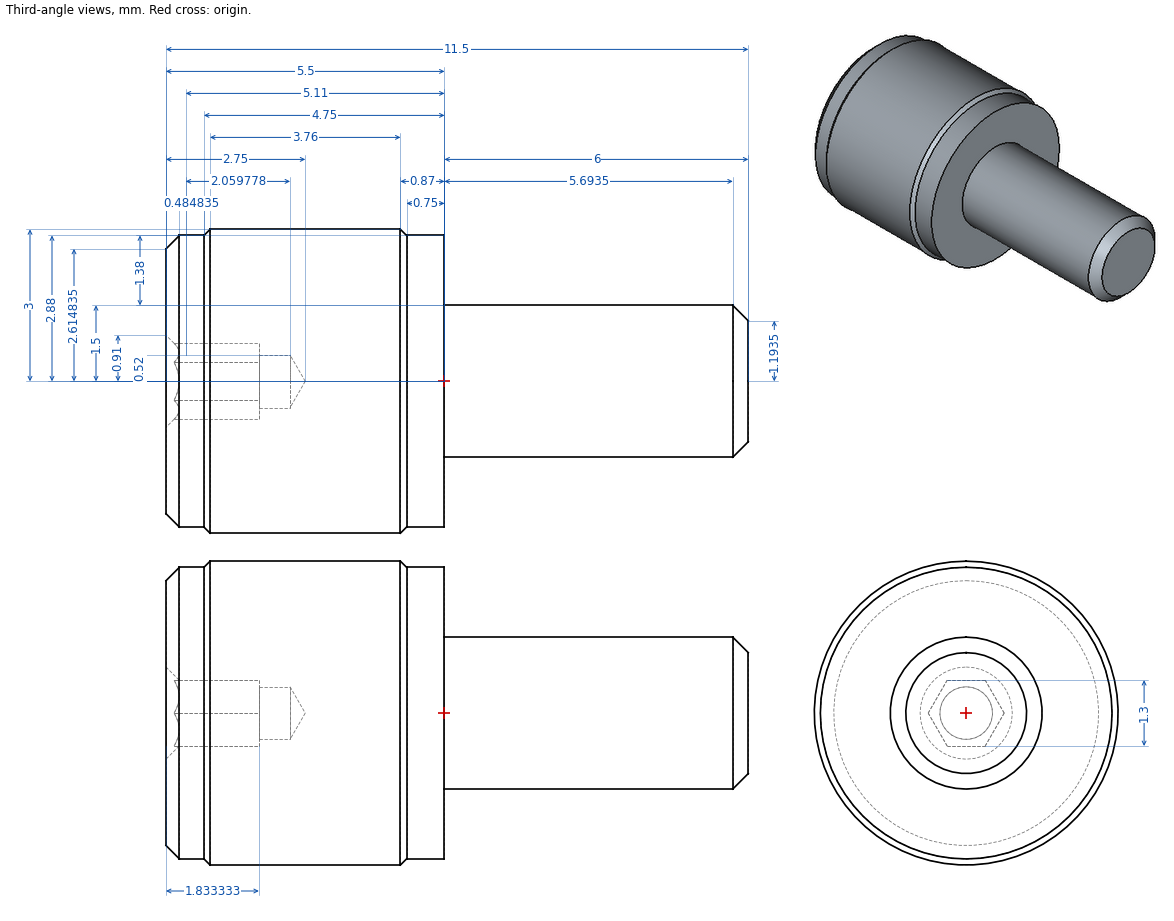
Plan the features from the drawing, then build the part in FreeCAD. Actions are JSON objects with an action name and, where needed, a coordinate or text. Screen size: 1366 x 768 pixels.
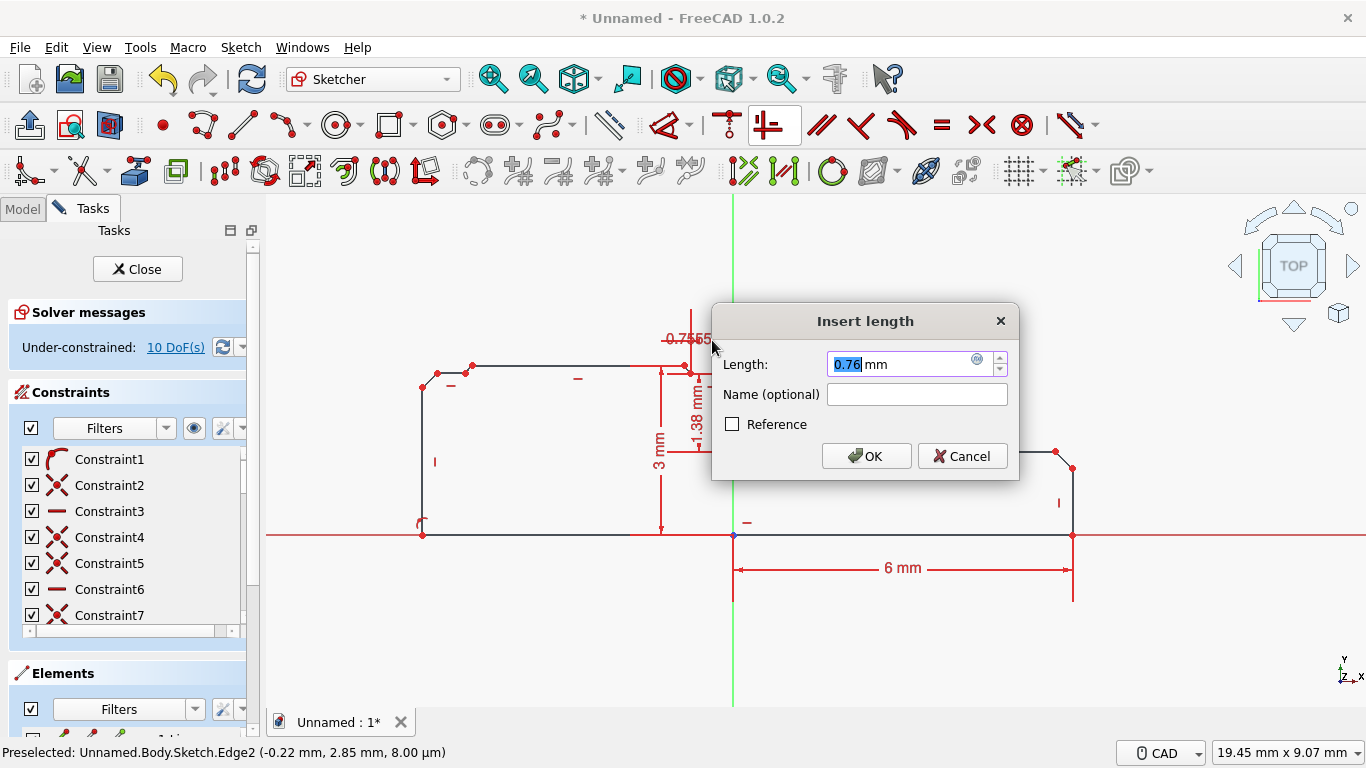
{"action": "type", "text": "0.75"}
{"action": "key", "text": "Return"}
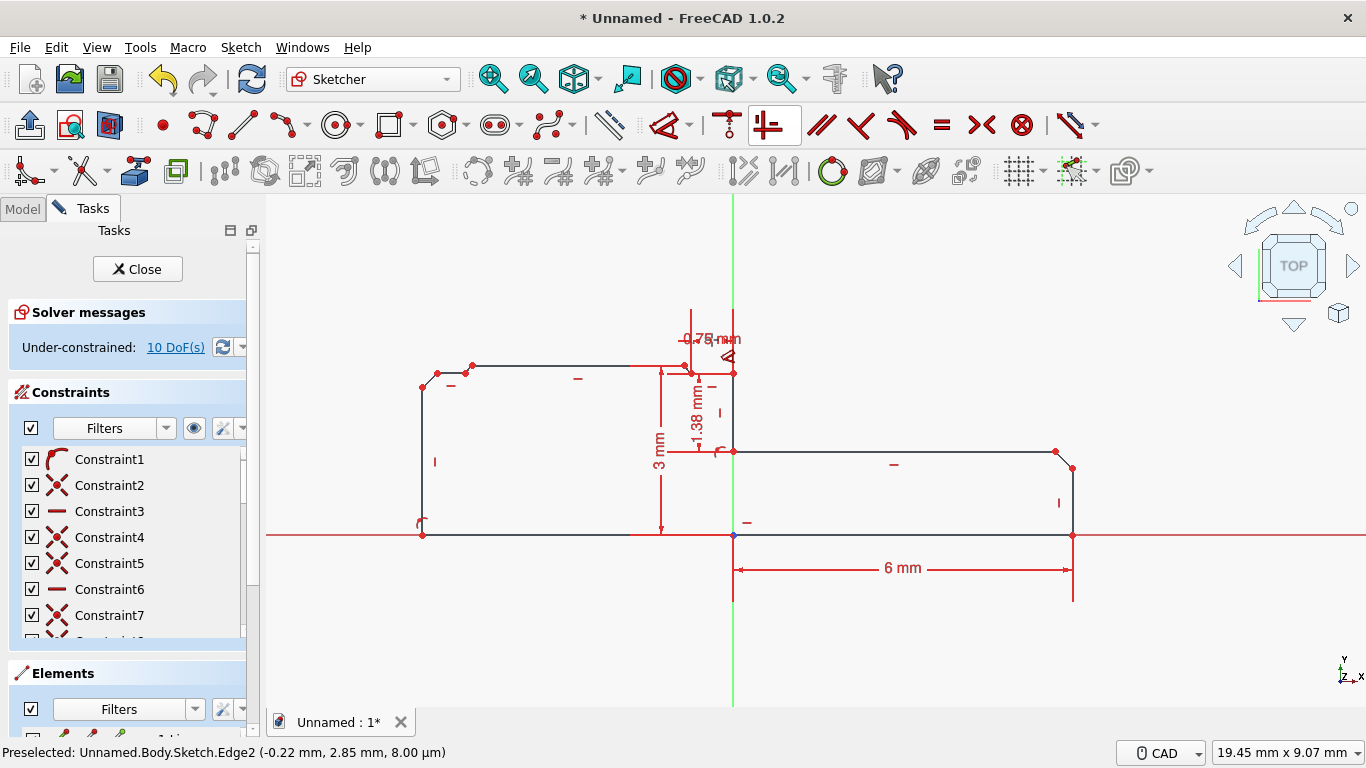
{"action": "left_click", "coordinate": [621, 366]}
{"action": "left_click", "coordinate": [578, 332]}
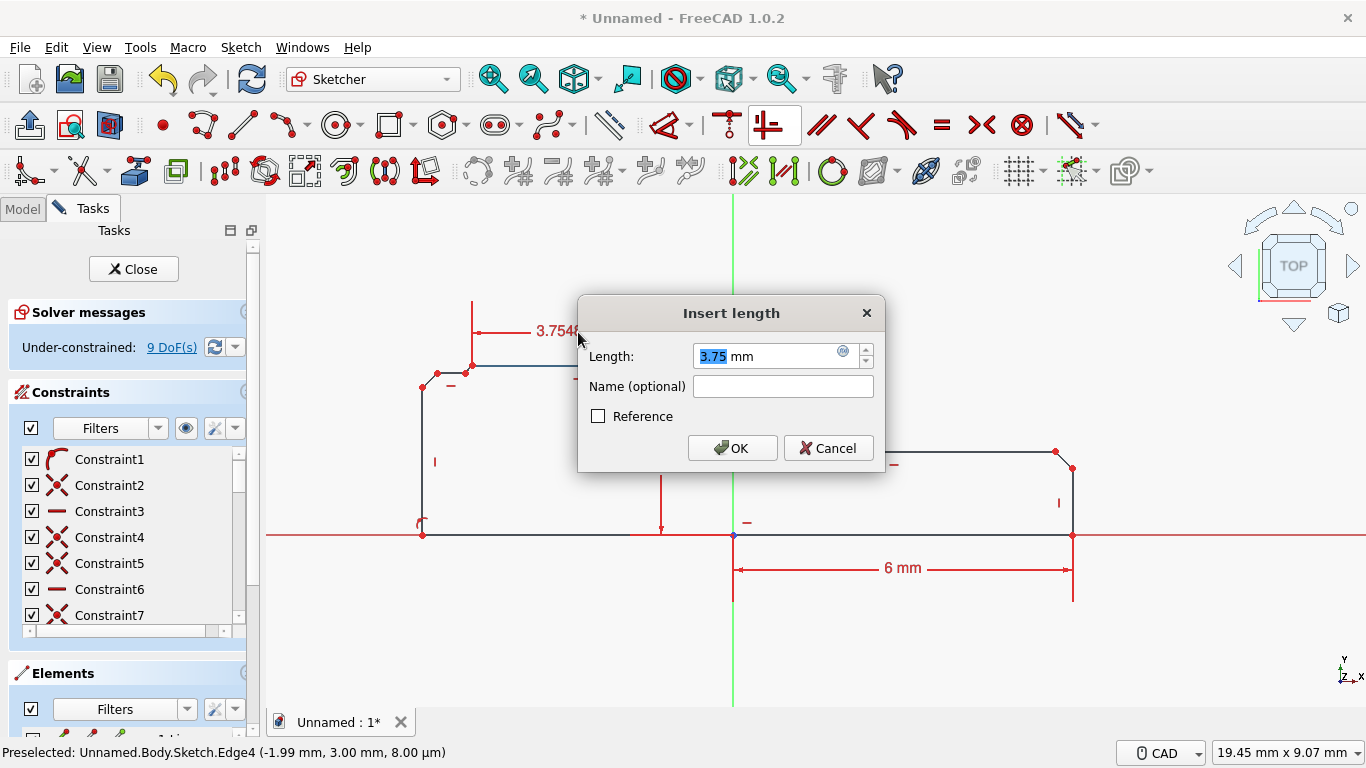
{"action": "type", "text": "3.76"}
{"action": "key", "text": "Return"}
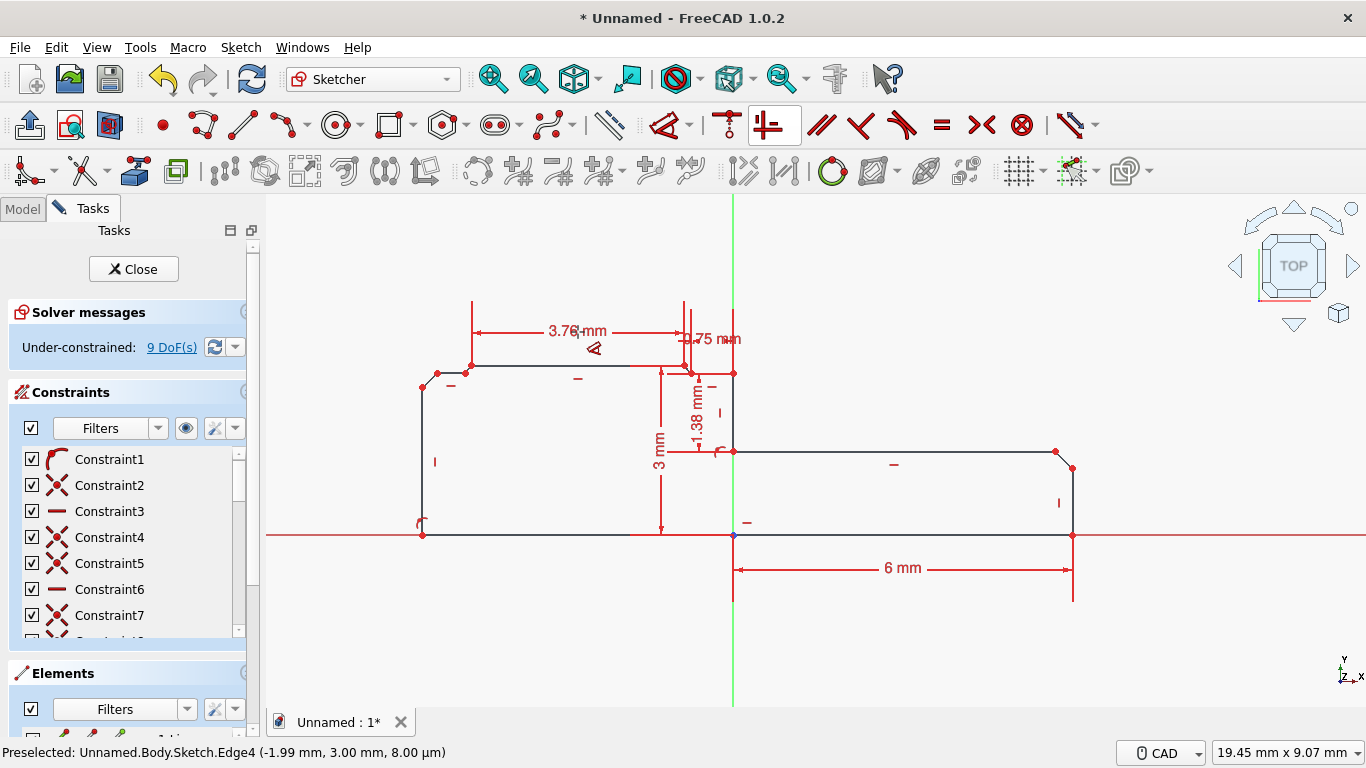
{"action": "left_click", "coordinate": [617, 535]}
{"action": "left_click", "coordinate": [748, 569]}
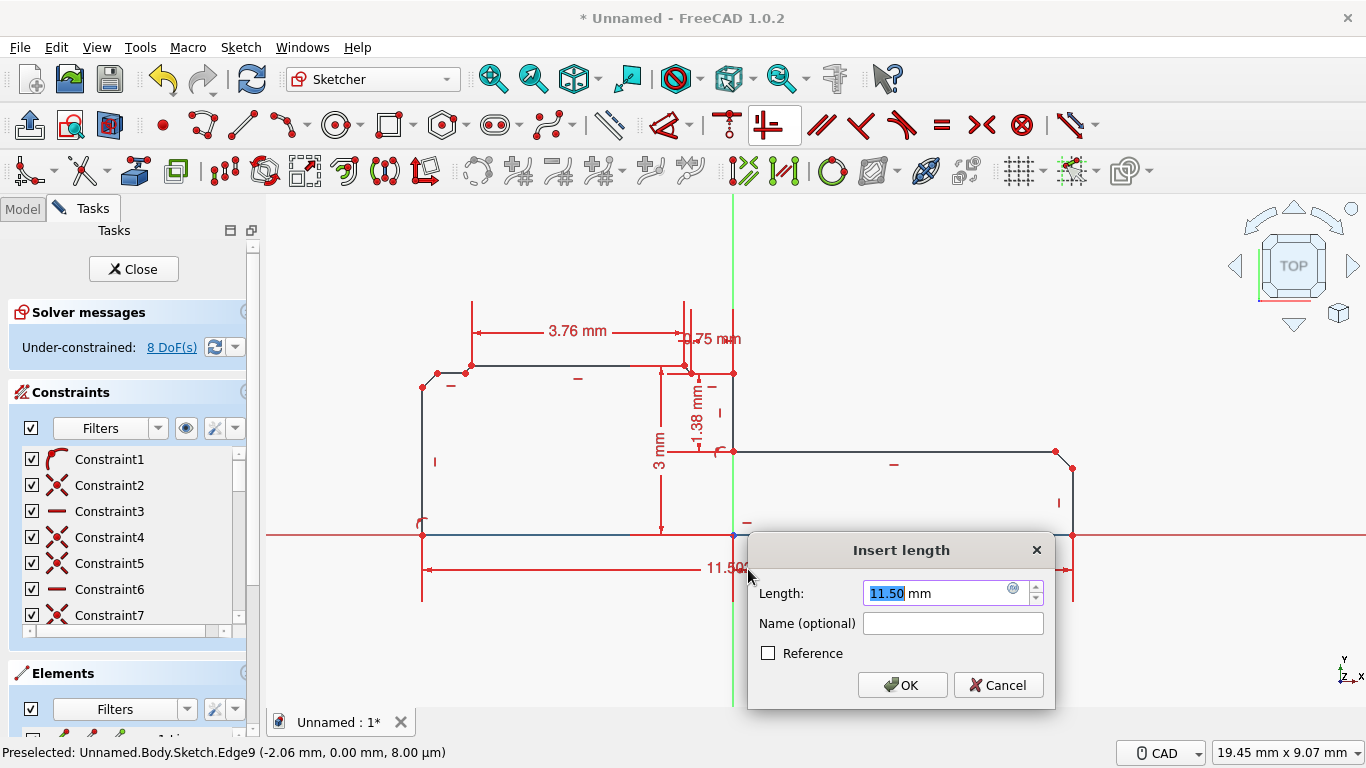
{"action": "type", "text": "11.5"}
{"action": "key", "text": "Return"}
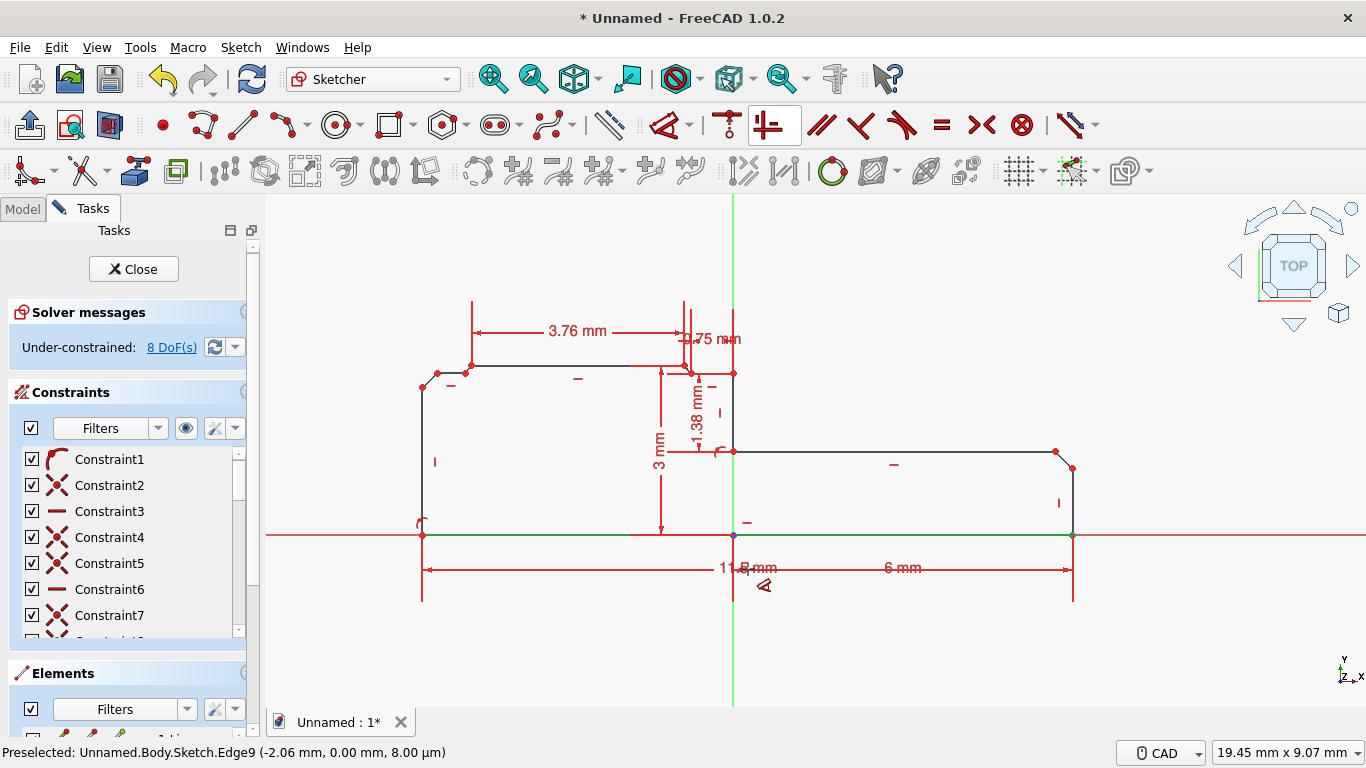
{"action": "left_click", "coordinate": [733, 452]}
{"action": "left_click", "coordinate": [699, 494]}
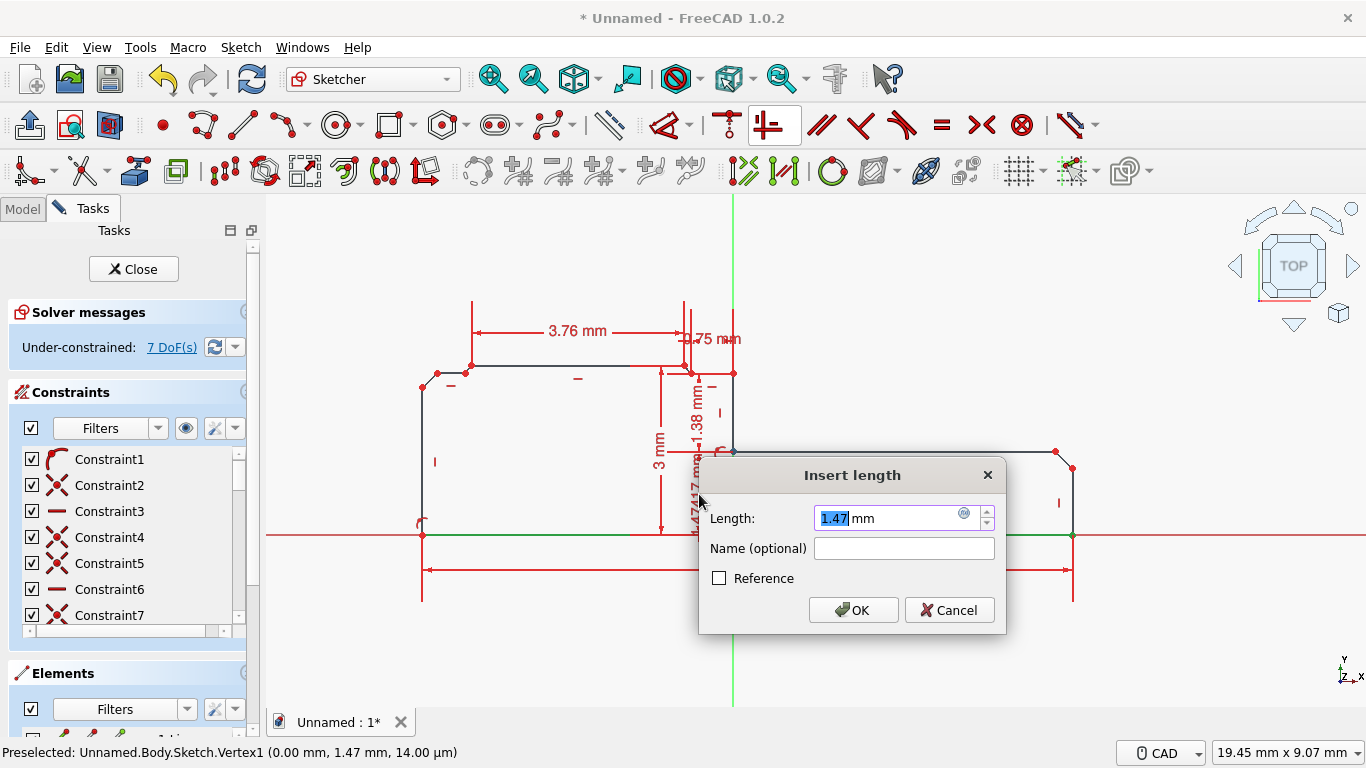
{"action": "type", "text": "1.5"}
{"action": "key", "text": "Return"}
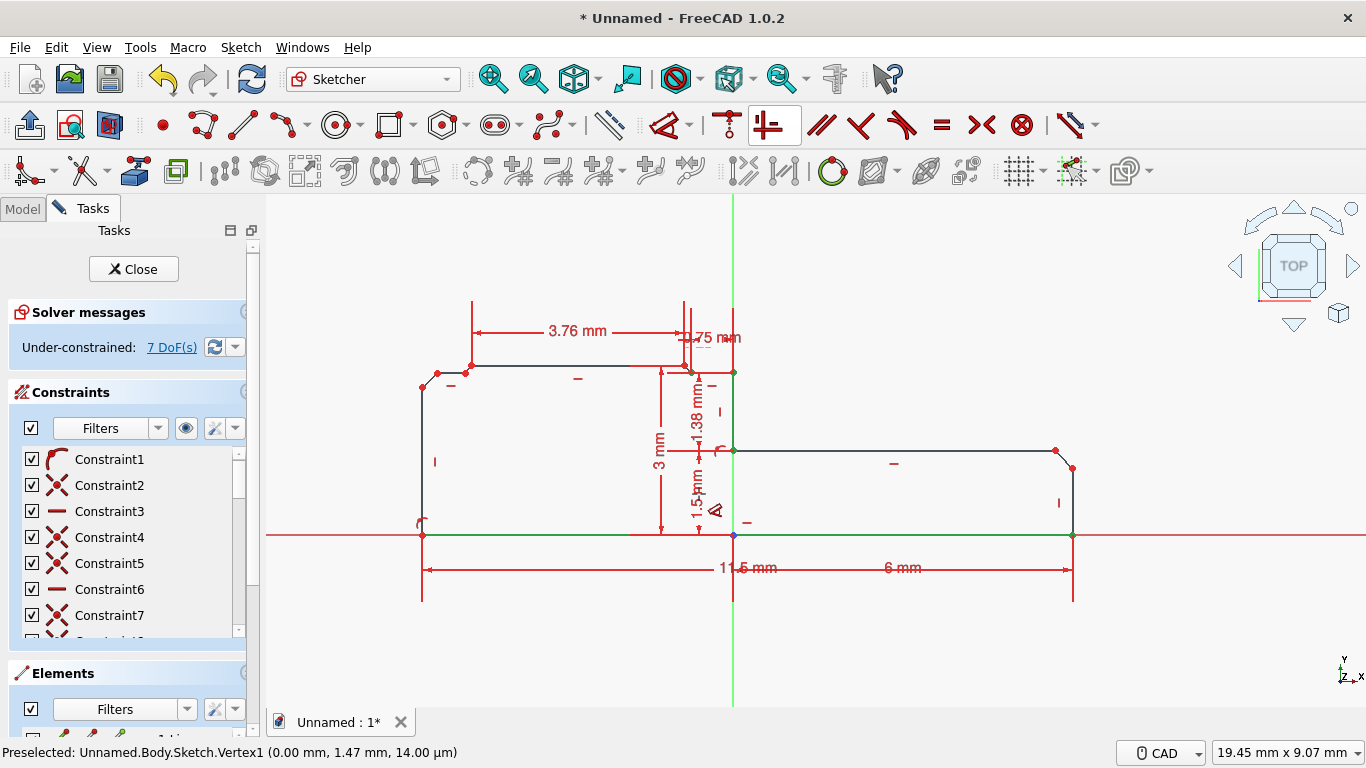
{"action": "scroll", "coordinate": [684, 366], "scroll_direction": "up", "scroll_amount": 2}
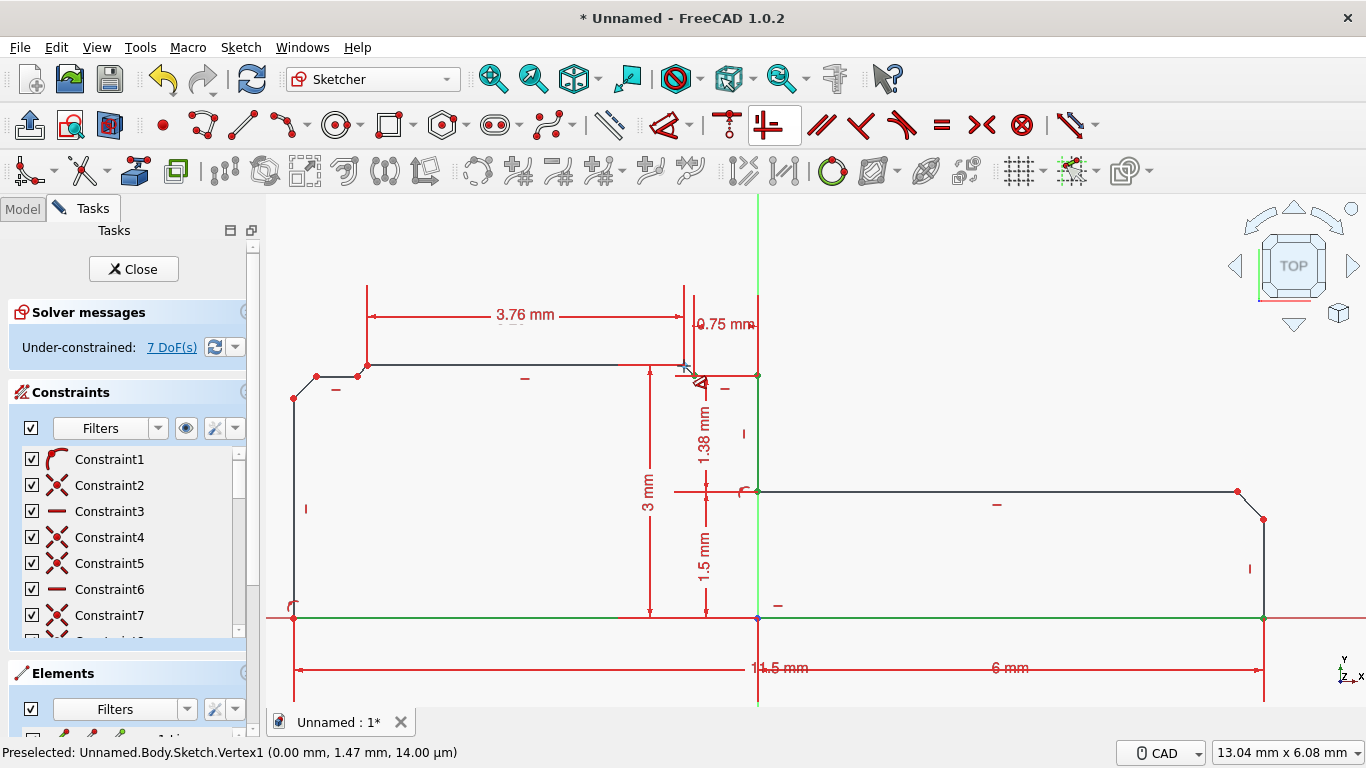
{"action": "left_click", "coordinate": [684, 365]}
{"action": "left_click", "coordinate": [704, 652]}